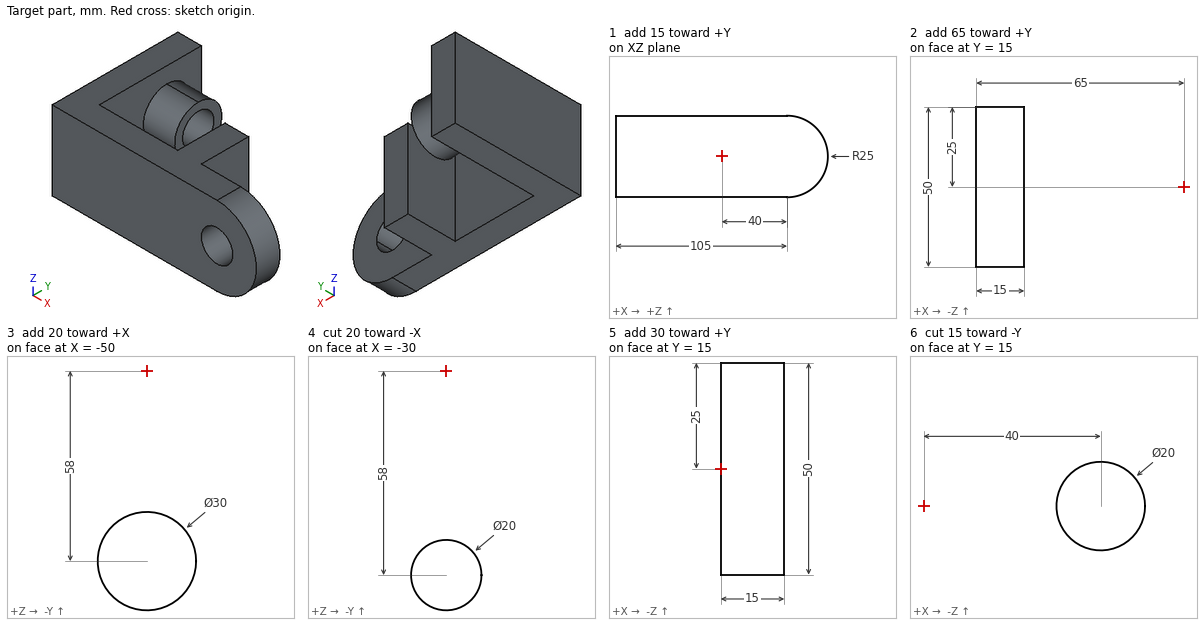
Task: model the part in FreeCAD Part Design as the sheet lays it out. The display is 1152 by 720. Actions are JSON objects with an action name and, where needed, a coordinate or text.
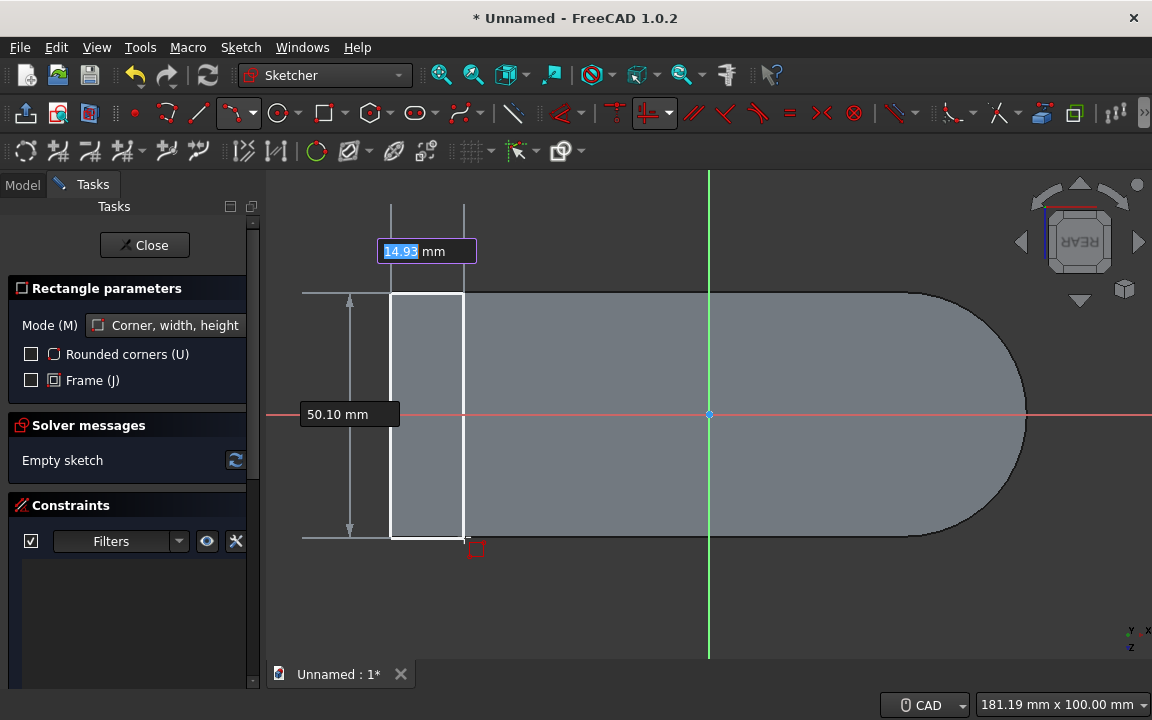
{"action": "type", "text": "15"}
{"action": "key", "text": "Tab"}
{"action": "type", "text": "50"}
{"action": "key", "text": "Return"}
{"action": "key", "text": "Escape"}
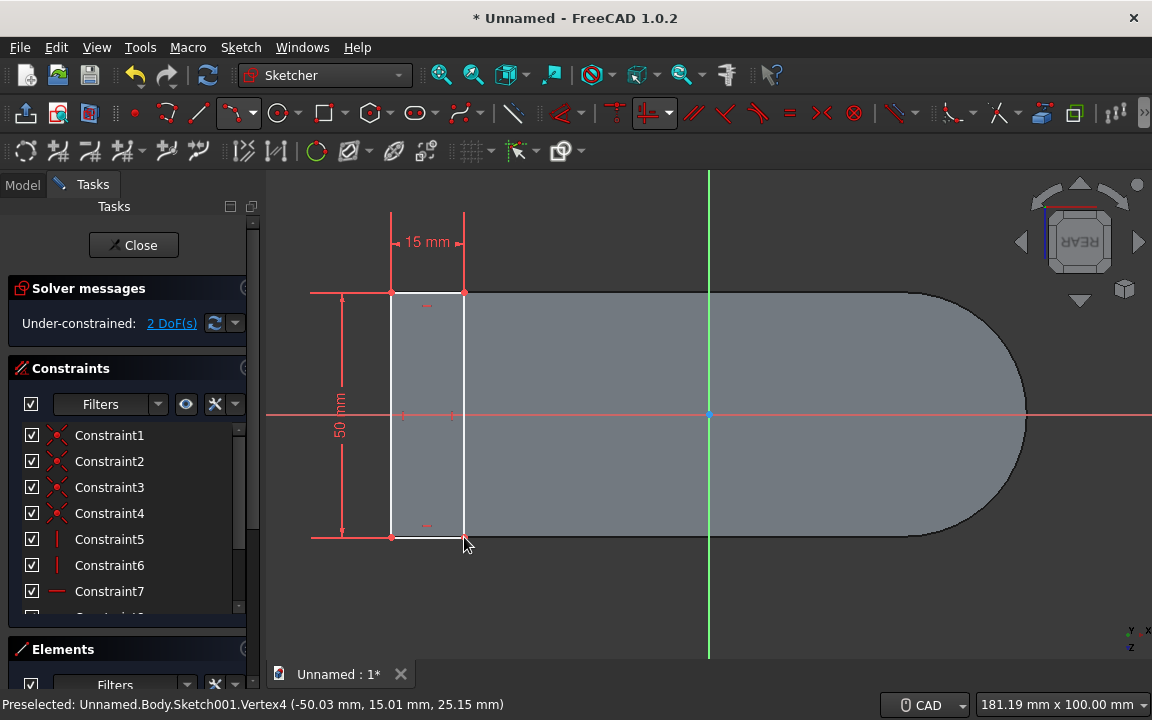
{"action": "left_click", "coordinate": [560, 114]}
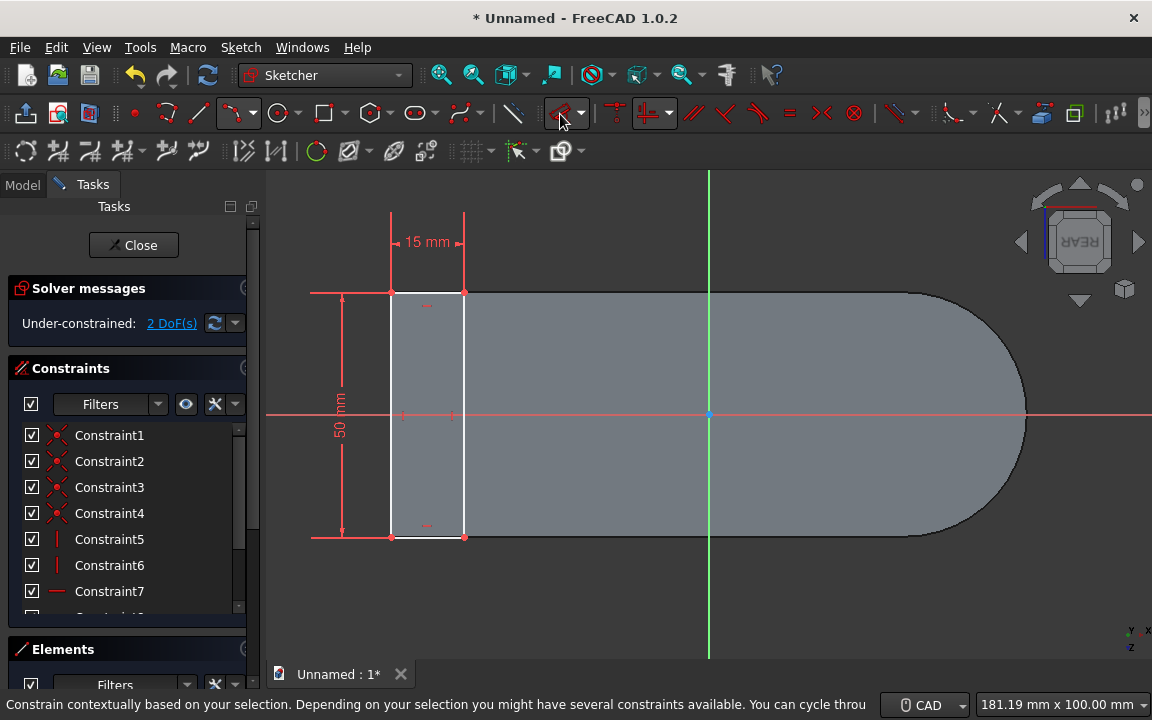
{"action": "left_click", "coordinate": [391, 293]}
{"action": "left_click", "coordinate": [550, 259]}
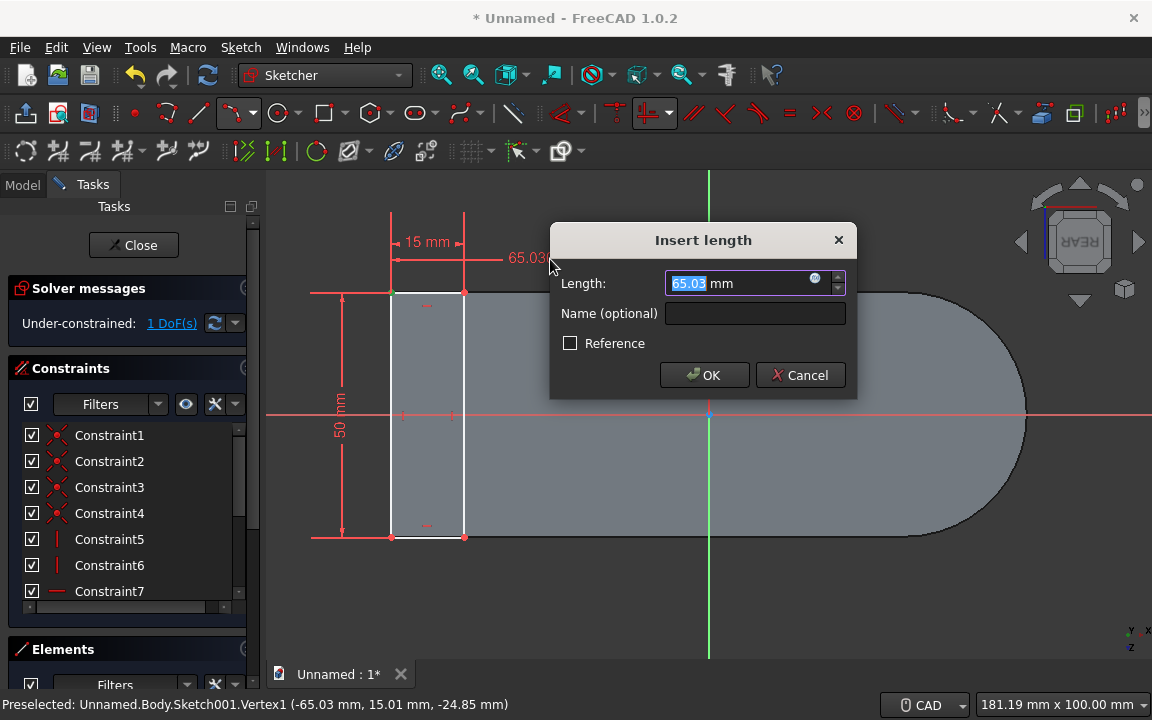
{"action": "type", "text": "65"}
{"action": "key", "text": "Return"}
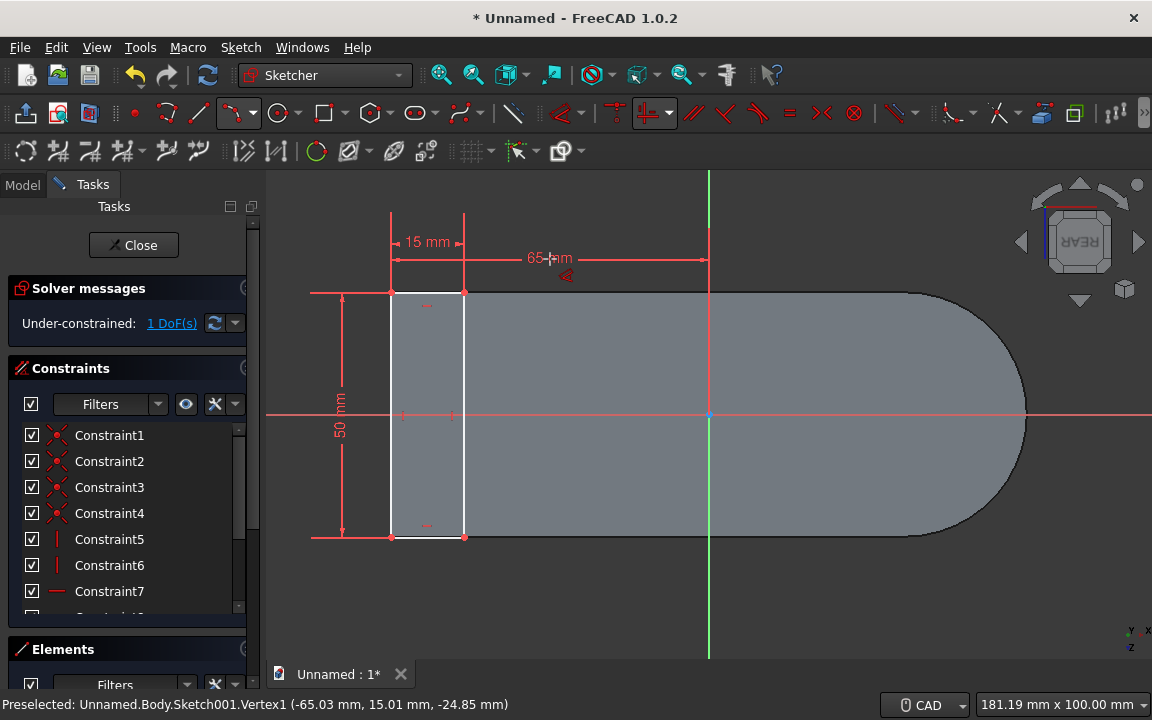
{"action": "left_click", "coordinate": [391, 293]}
{"action": "left_click", "coordinate": [743, 354]}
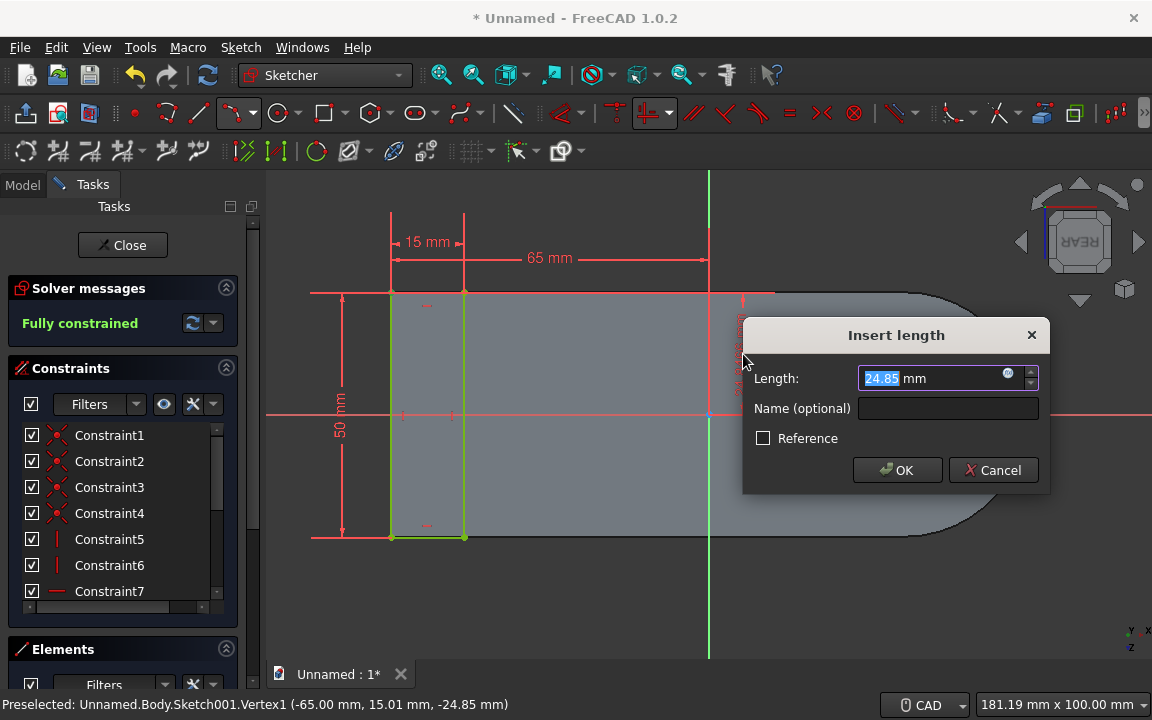
{"action": "type", "text": "25"}
{"action": "key", "text": "Return"}
{"action": "key", "text": "Escape"}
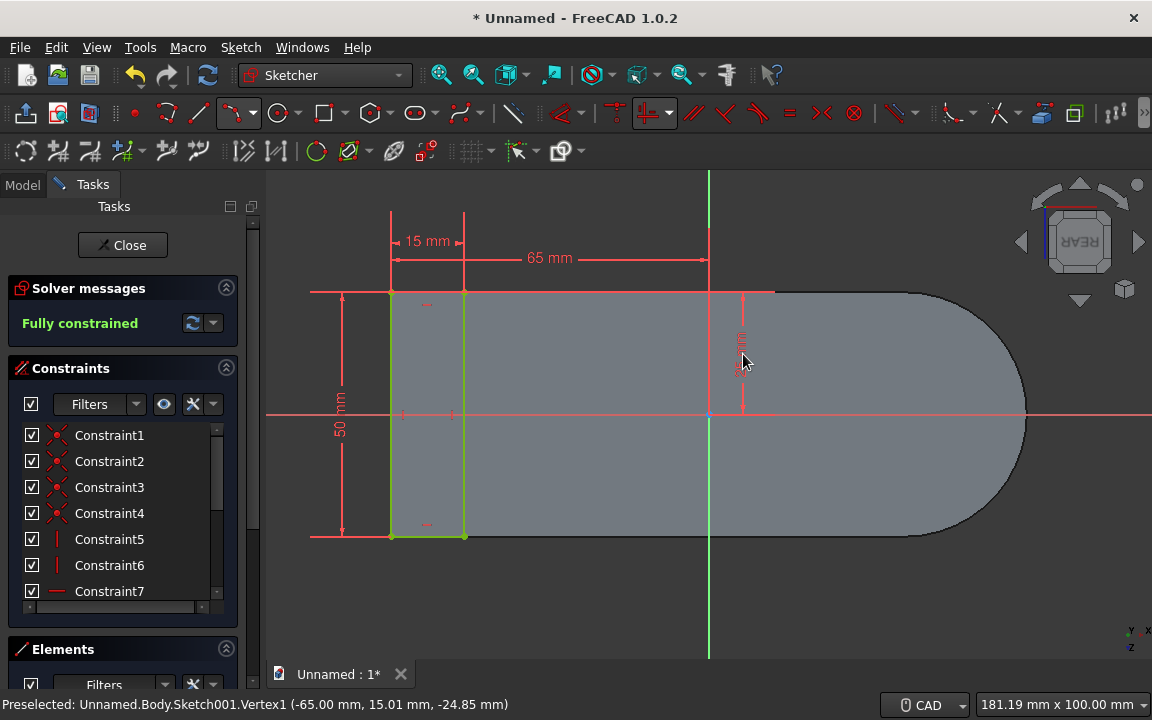
{"action": "left_click", "coordinate": [123, 245]}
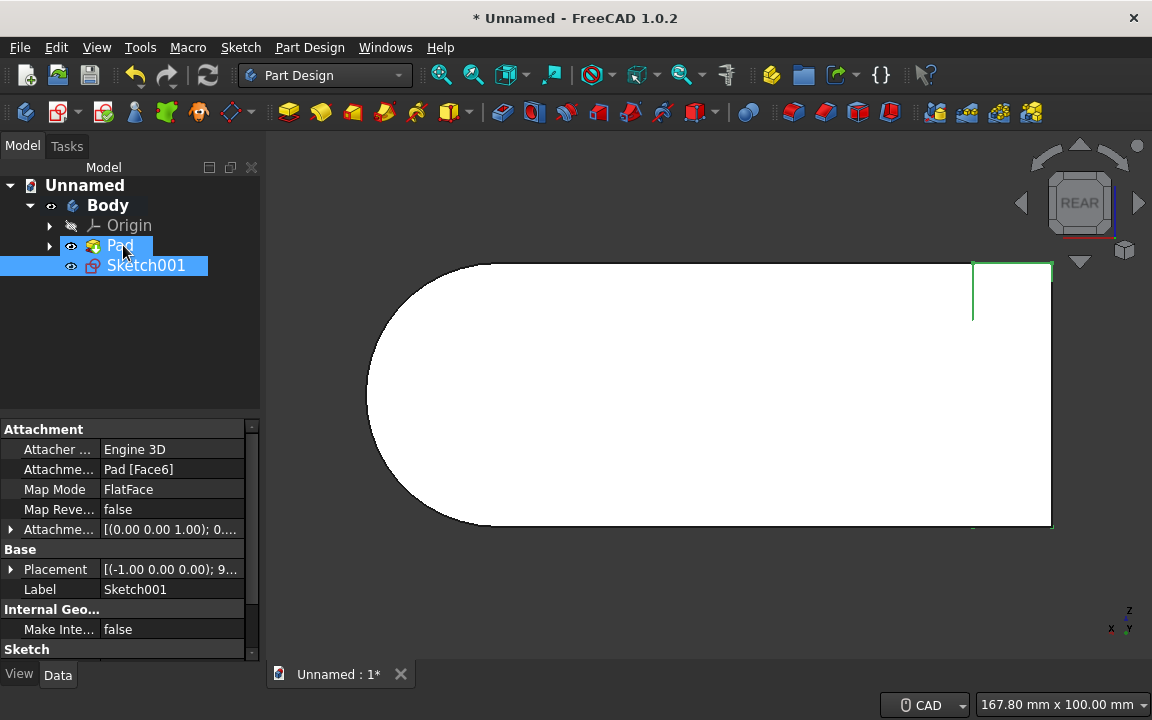
{"action": "left_click", "coordinate": [290, 112]}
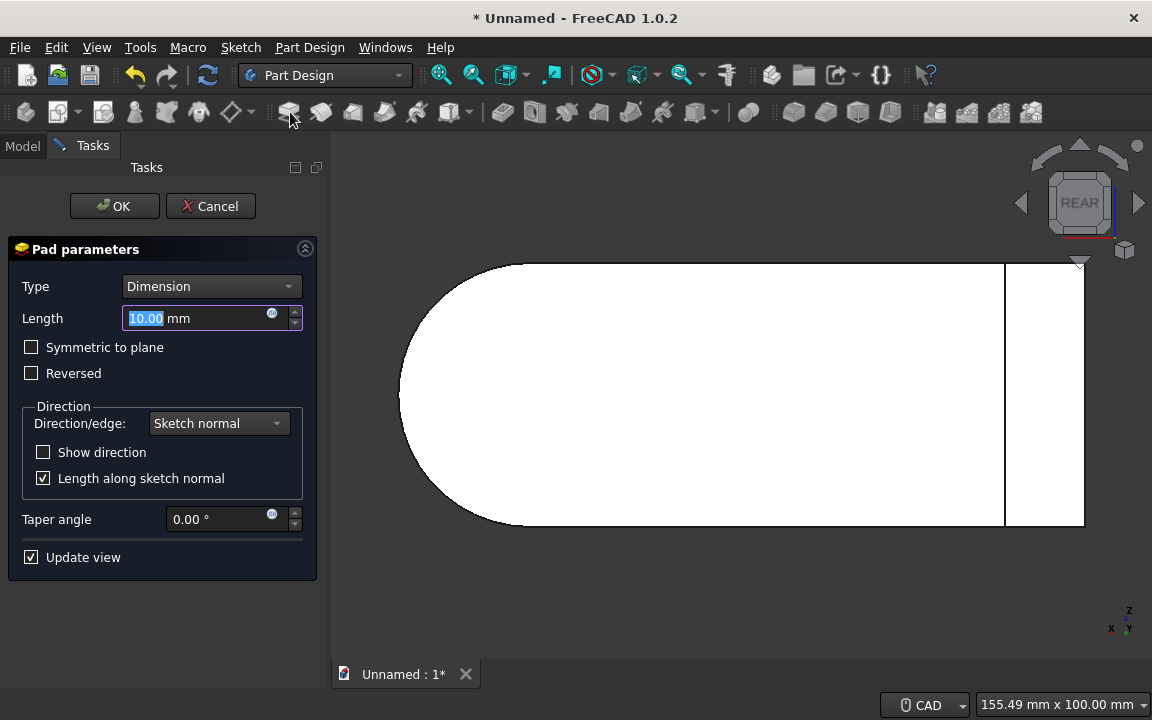
{"action": "type", "text": "65"}
{"action": "key", "text": "Tab"}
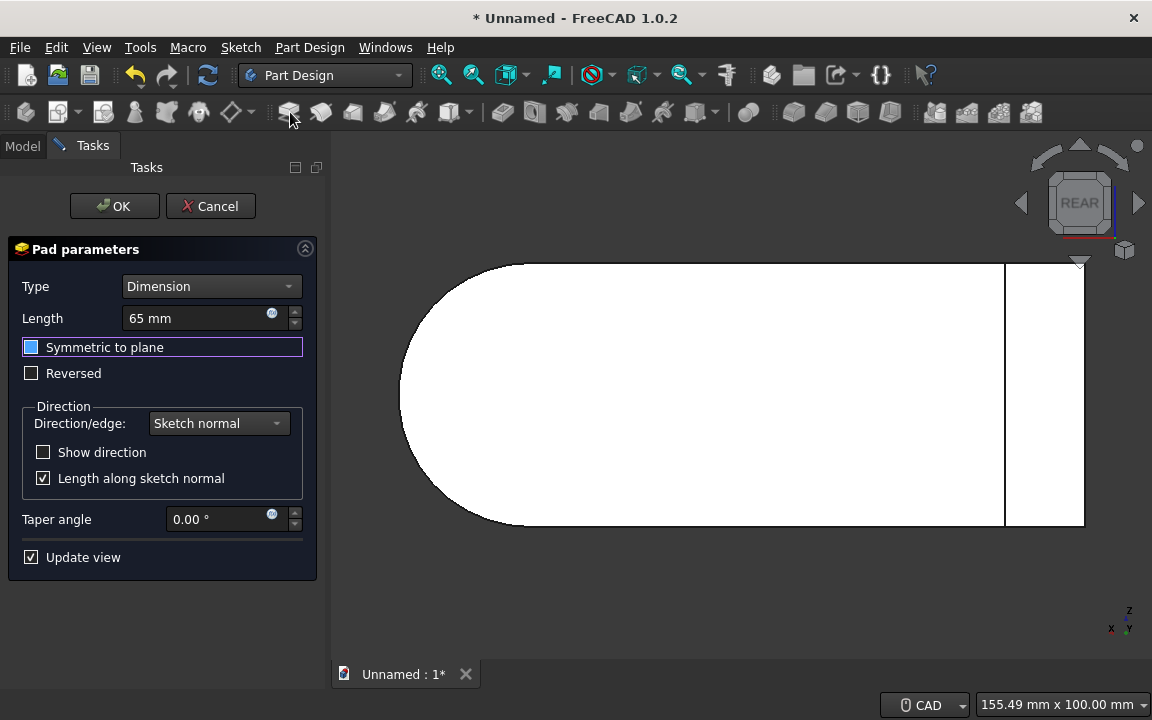
{"action": "left_click", "coordinate": [115, 206]}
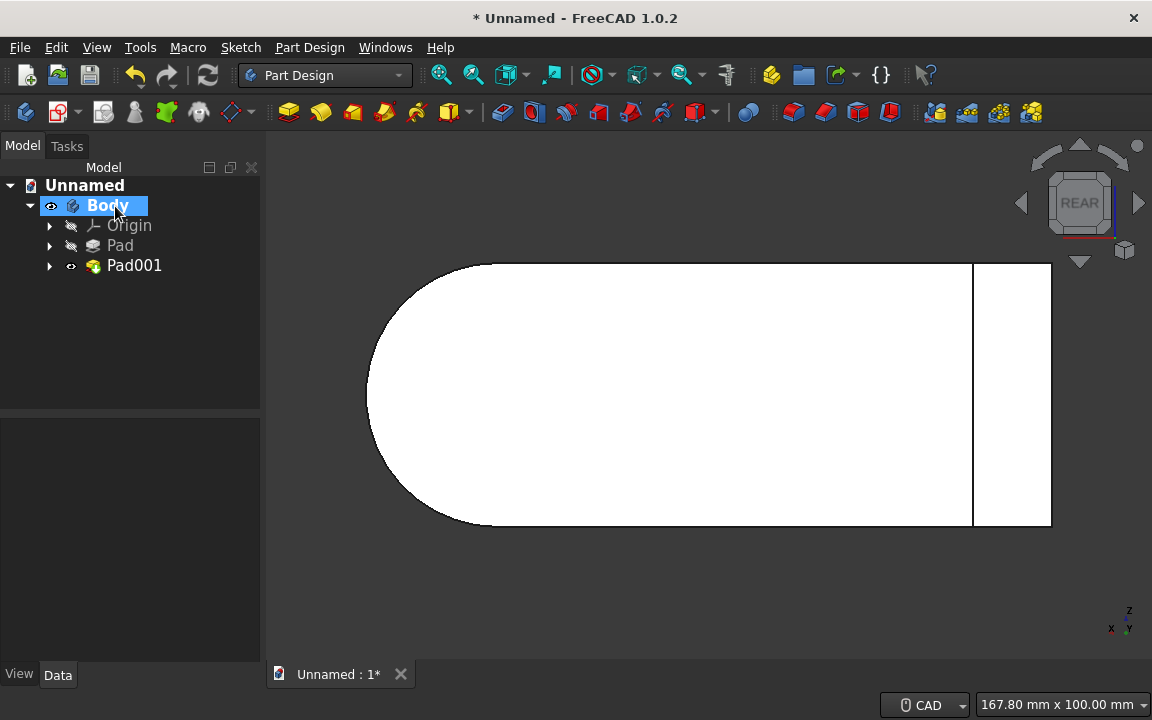
{"action": "key", "text": "0"}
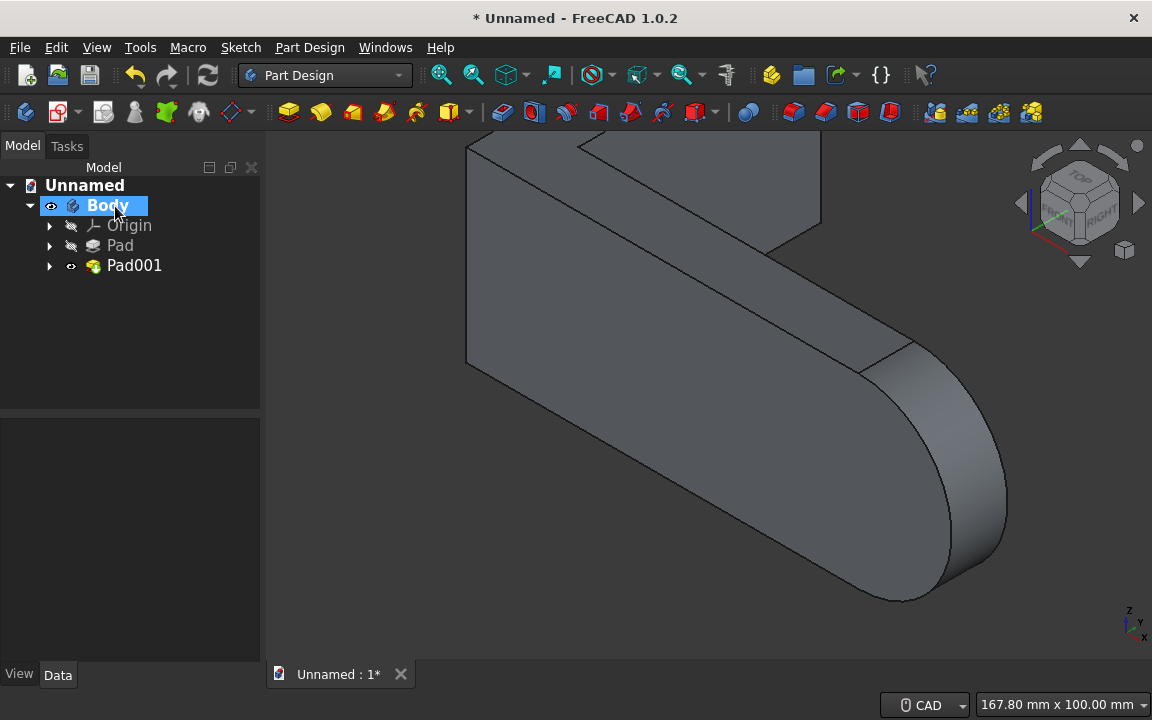
{"action": "left_click", "coordinate": [442, 76]}